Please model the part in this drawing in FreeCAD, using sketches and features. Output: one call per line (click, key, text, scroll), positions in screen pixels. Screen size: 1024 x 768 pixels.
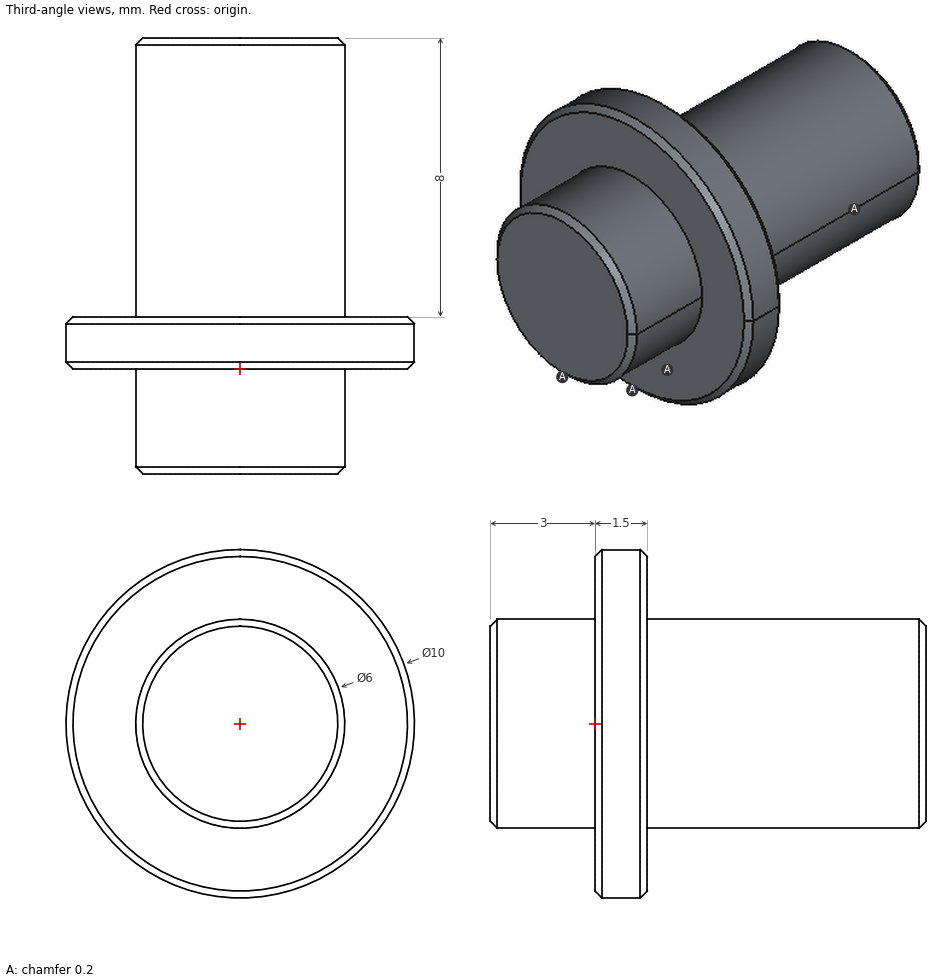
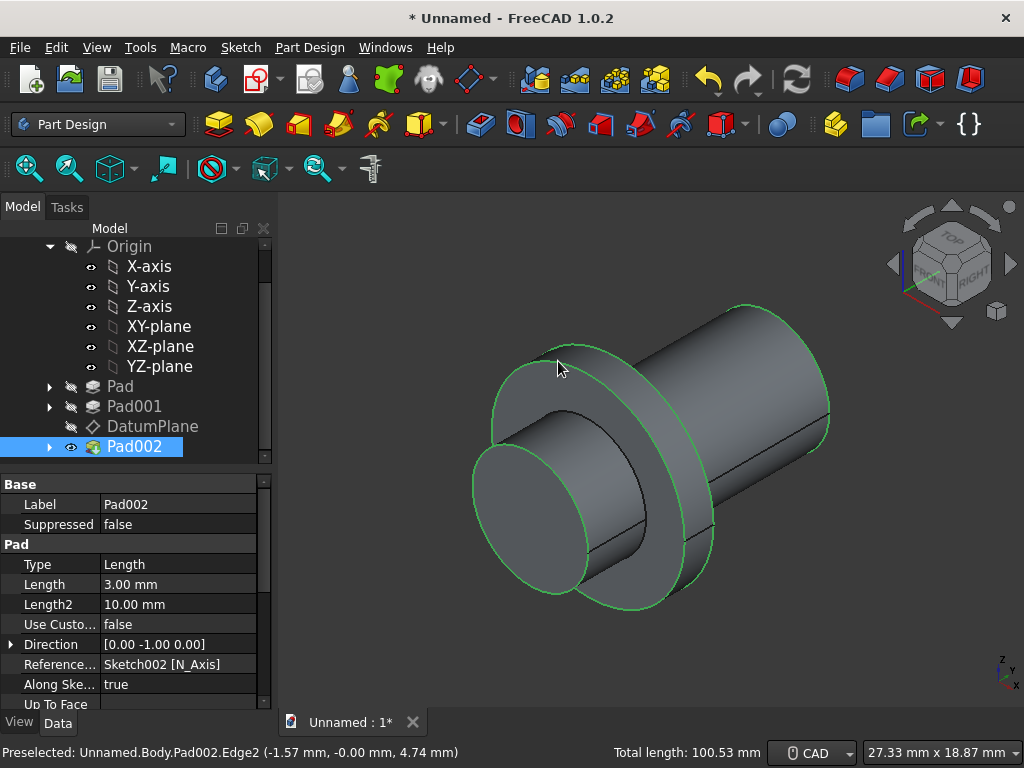
click(890, 80)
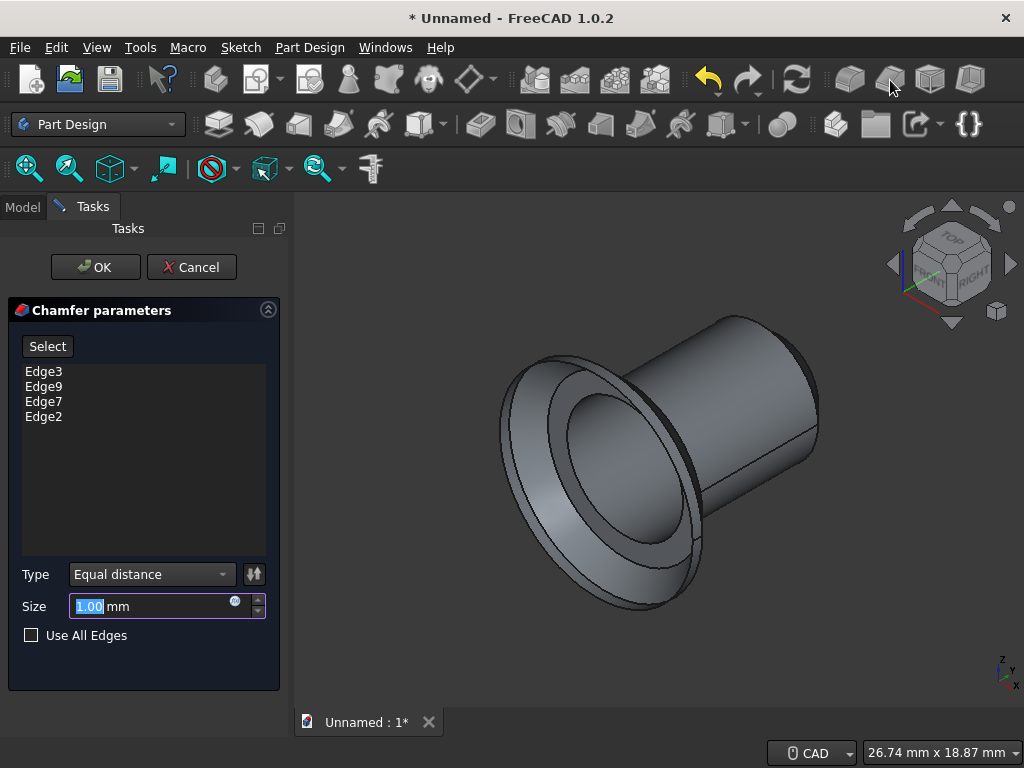
text(0.2)
key(Tab)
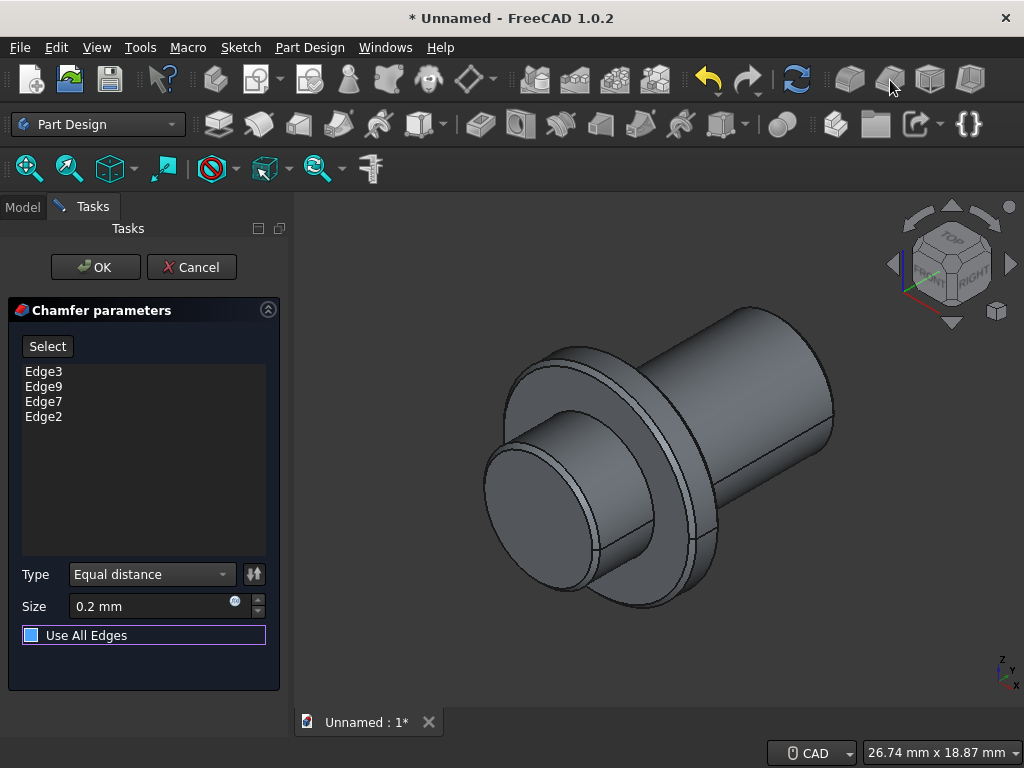
click(96, 267)